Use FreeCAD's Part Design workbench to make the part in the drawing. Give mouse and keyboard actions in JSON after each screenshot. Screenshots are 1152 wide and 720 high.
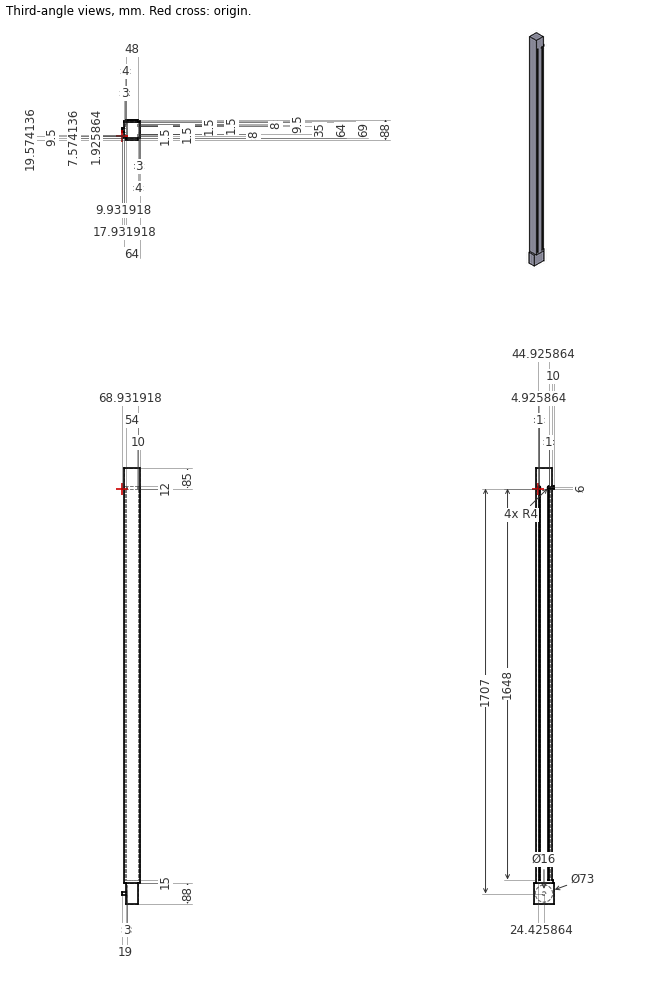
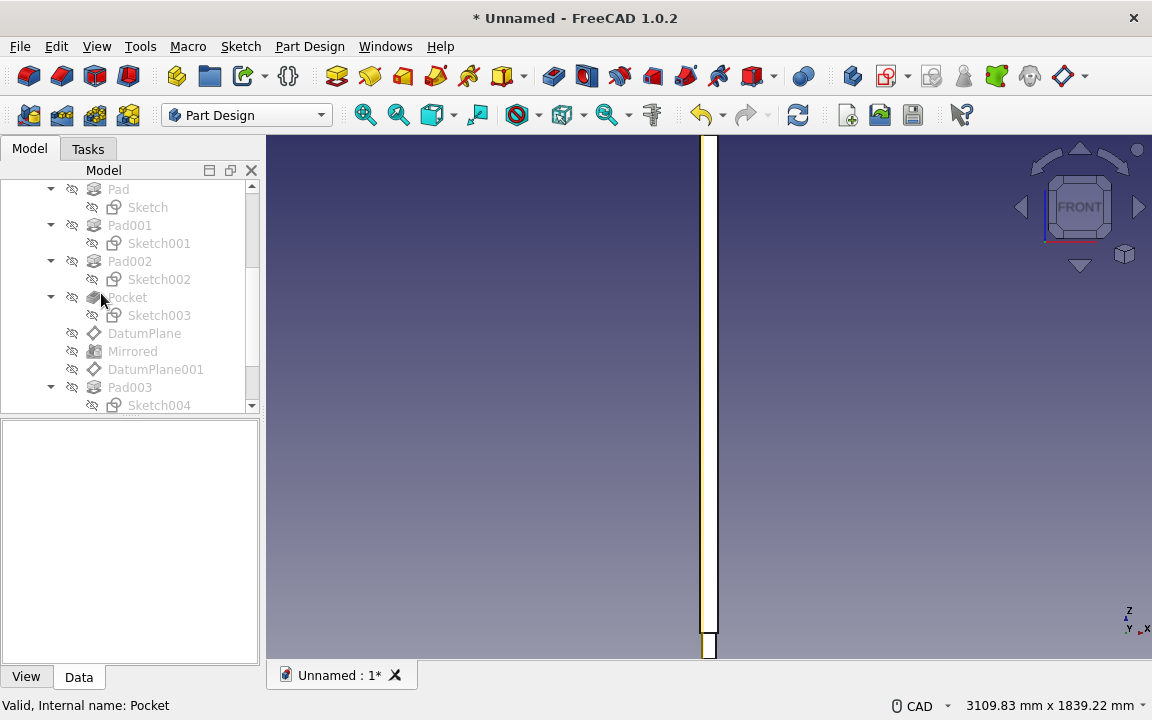
{"action": "scroll", "coordinate": [141, 293], "scroll_direction": "up", "scroll_amount": 15}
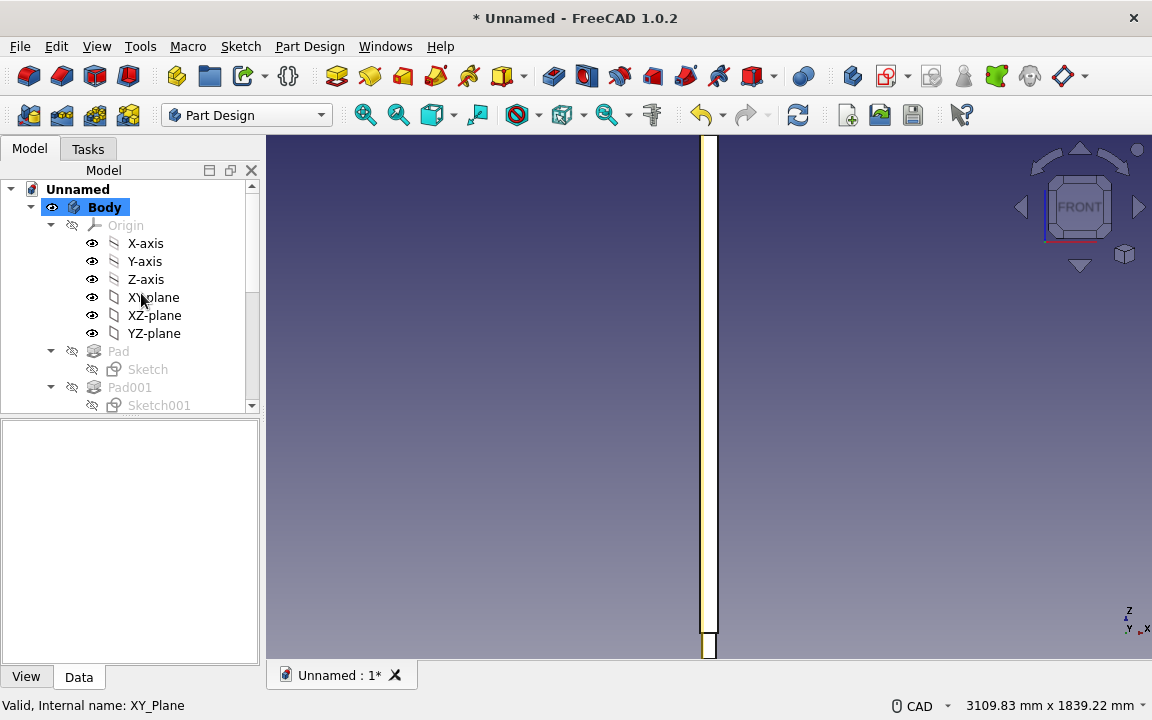
{"action": "scroll", "coordinate": [101, 293], "scroll_direction": "down", "scroll_amount": 6}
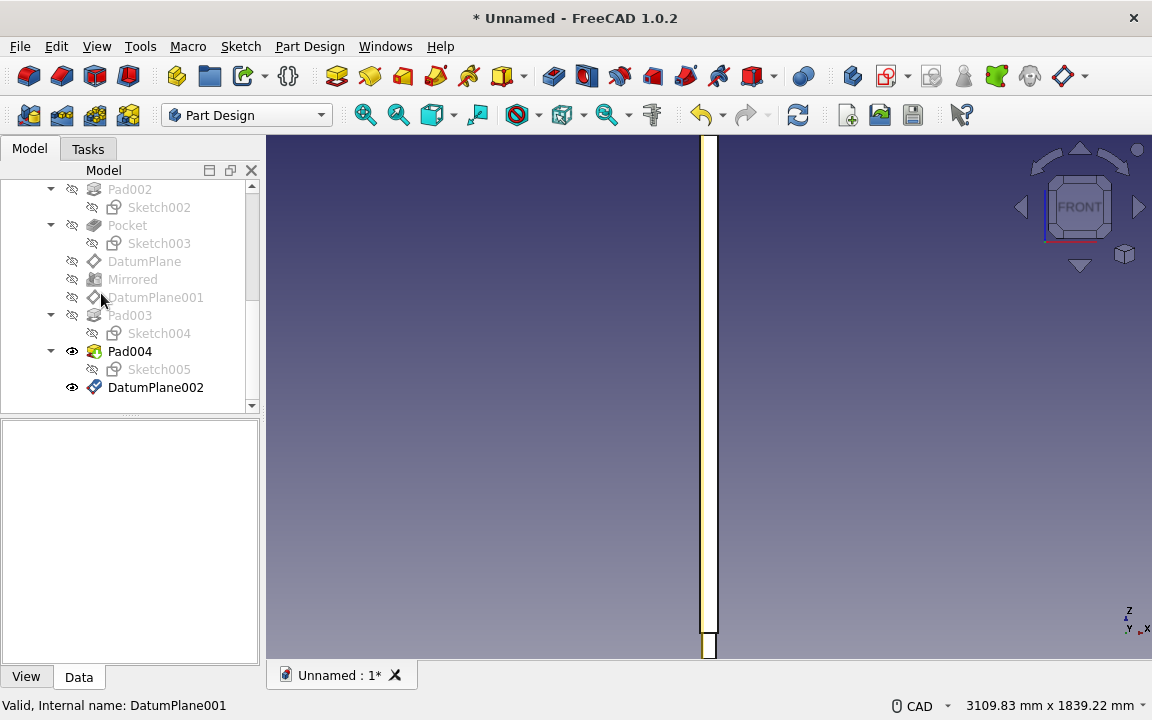
{"action": "left_click", "coordinate": [117, 387]}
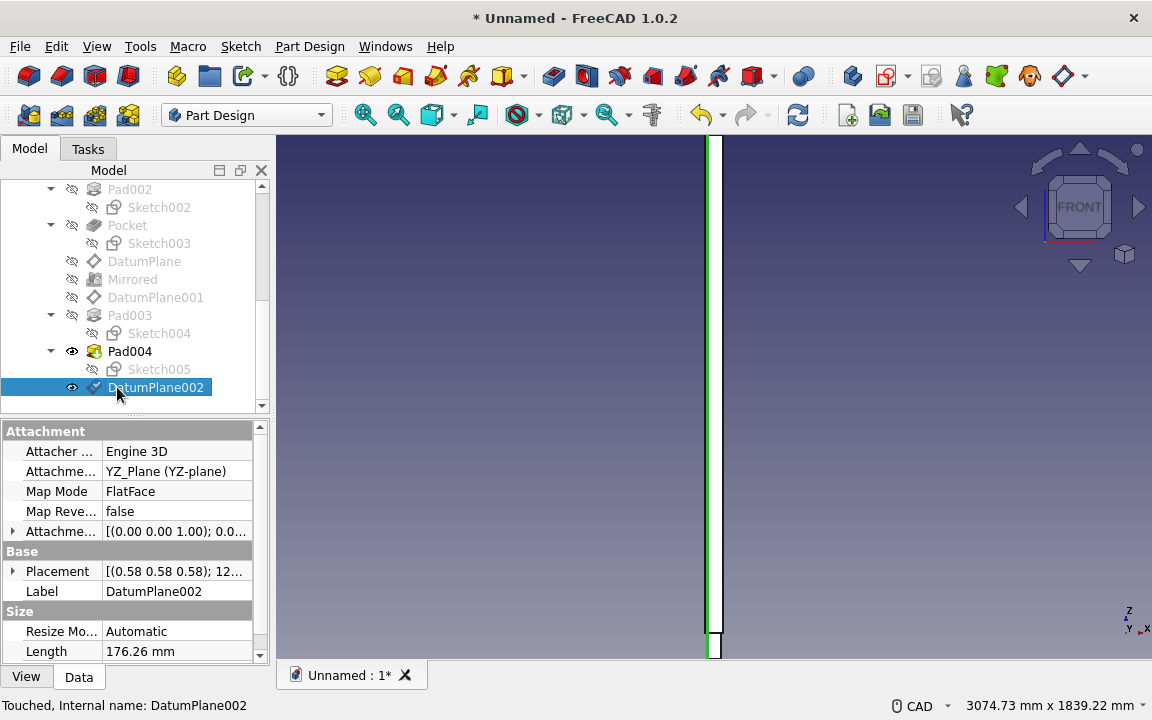
{"action": "left_click", "coordinate": [886, 76]}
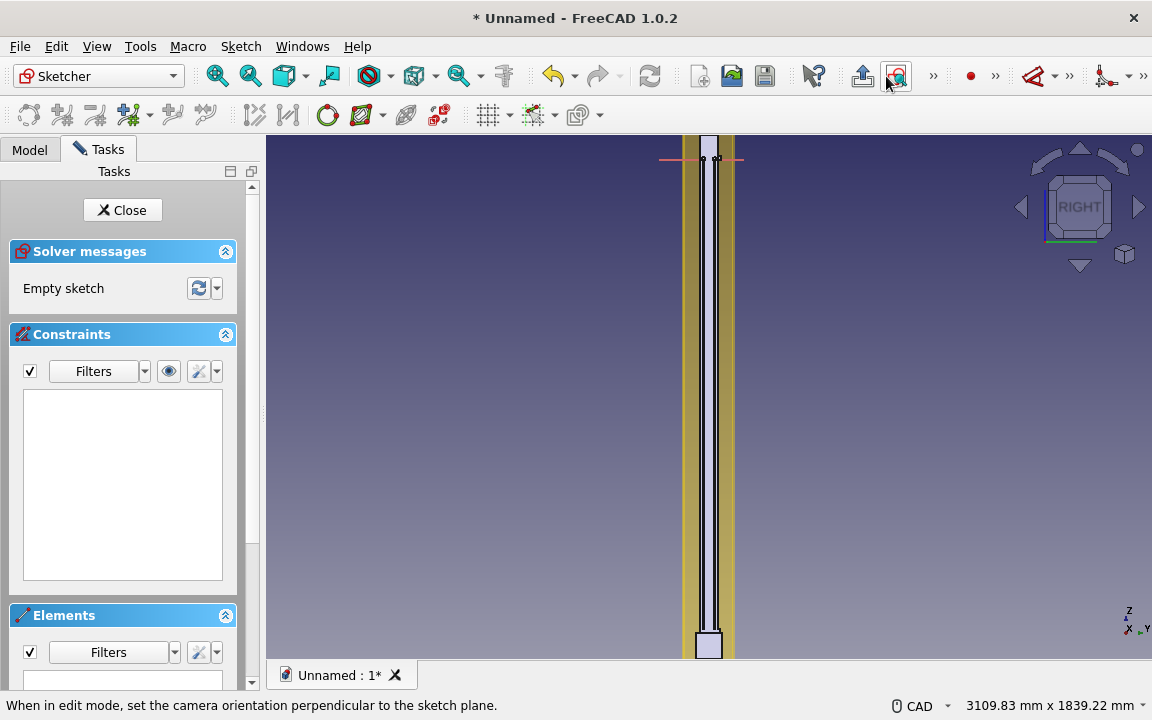
{"action": "key", "text": "q s"}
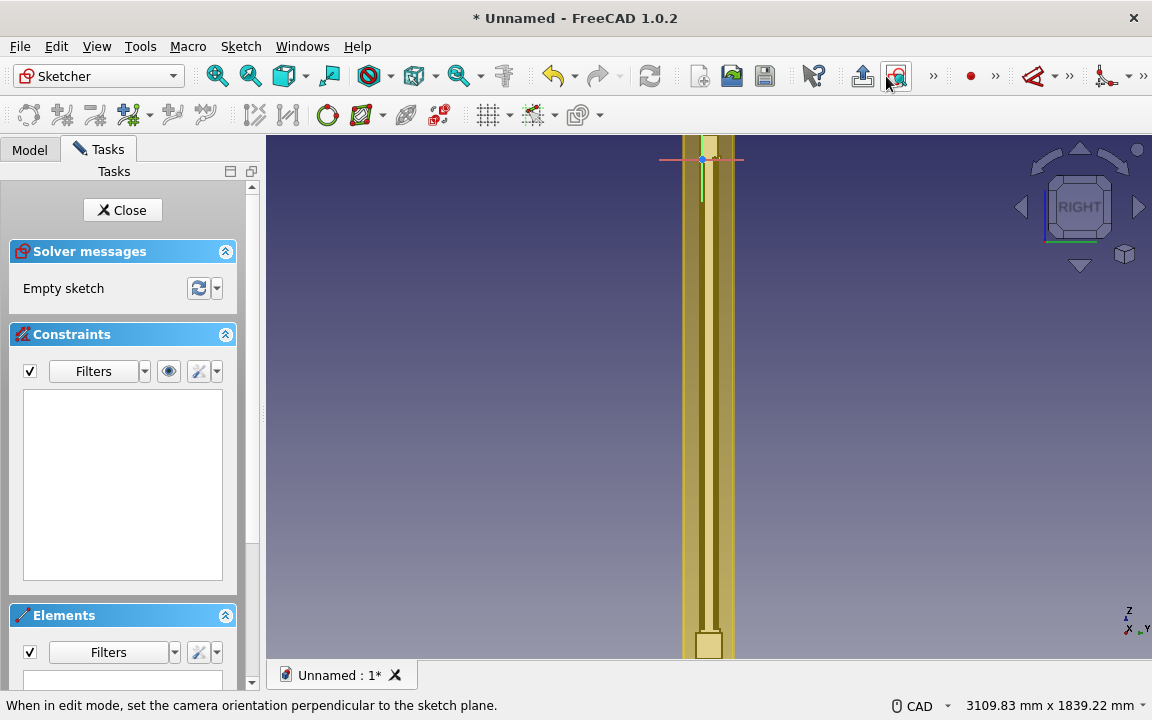
{"action": "scroll", "coordinate": [640, 397], "scroll_direction": "down", "scroll_amount": 5}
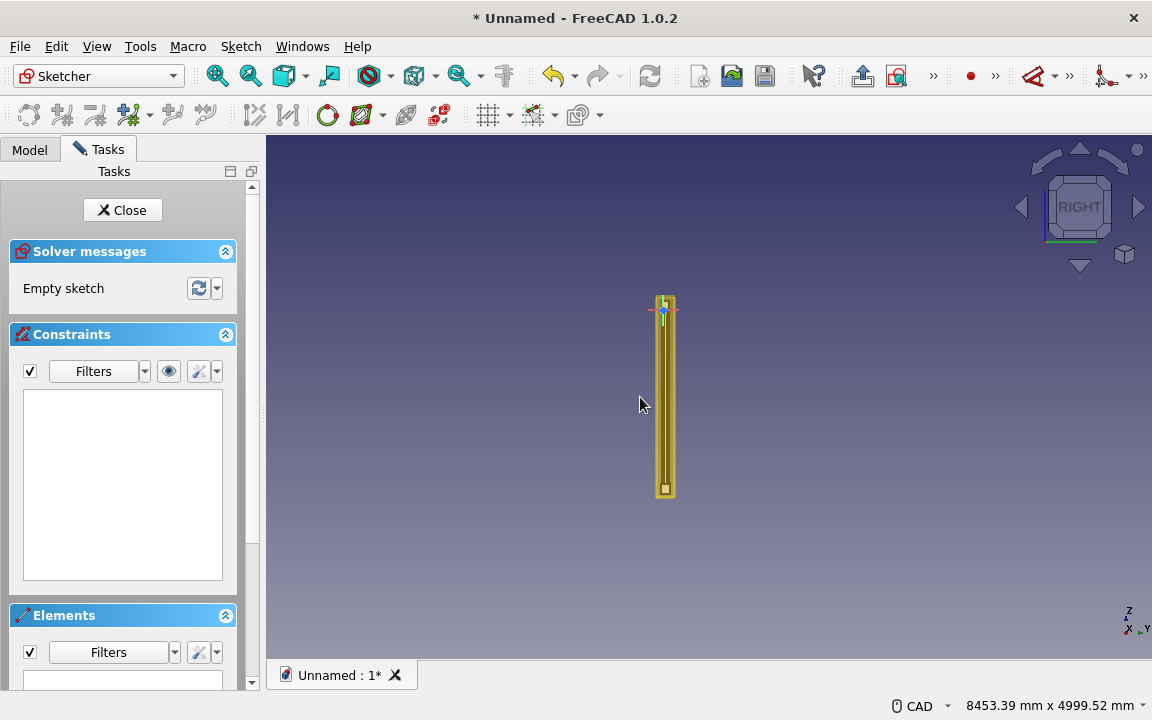
{"action": "scroll", "coordinate": [667, 494], "scroll_direction": "up", "scroll_amount": 15}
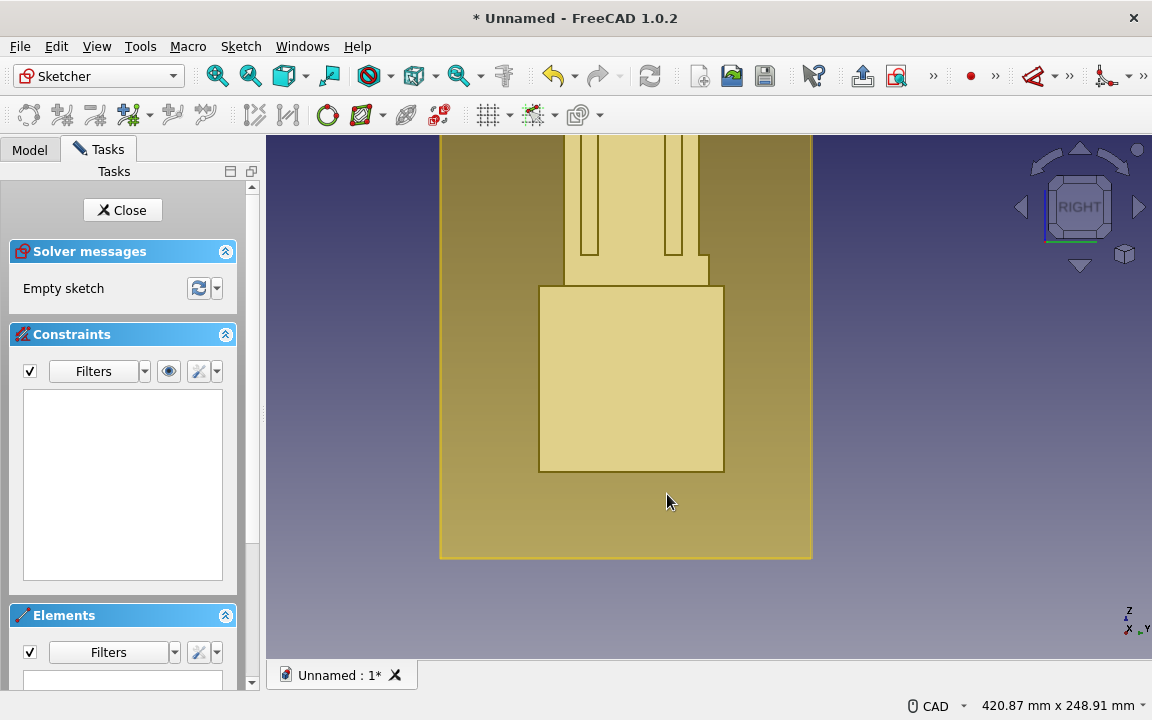
{"action": "scroll", "coordinate": [624, 364], "scroll_direction": "up", "scroll_amount": 4}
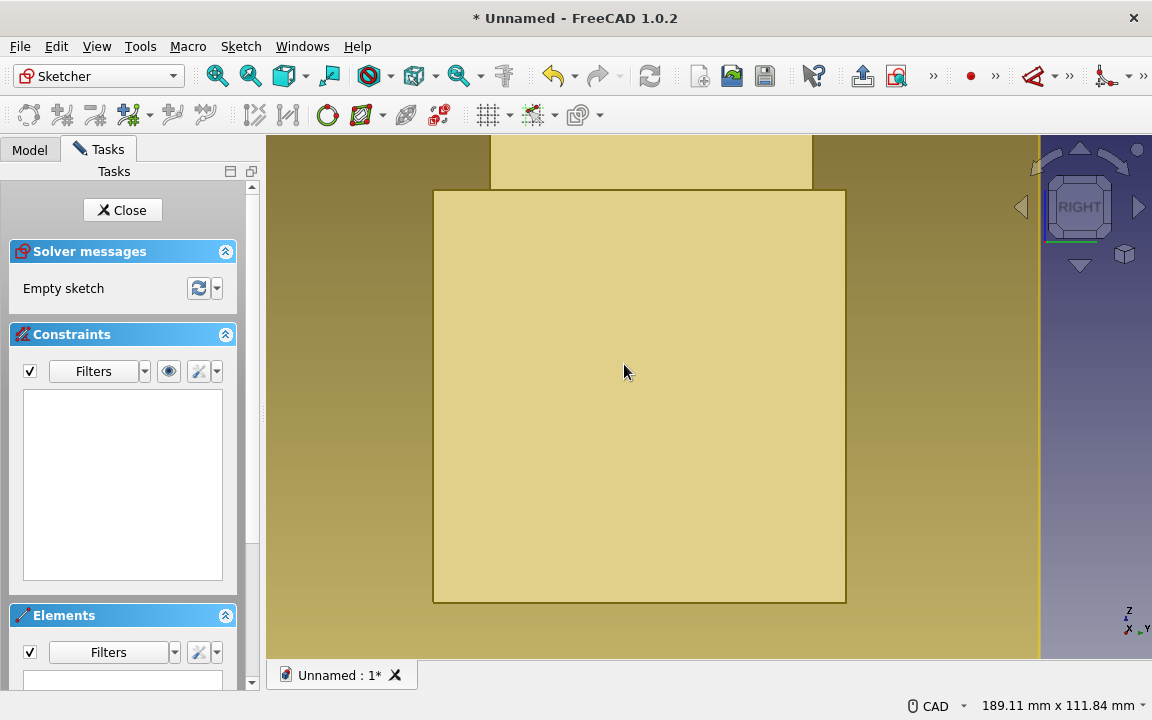
{"action": "key", "text": "g c"}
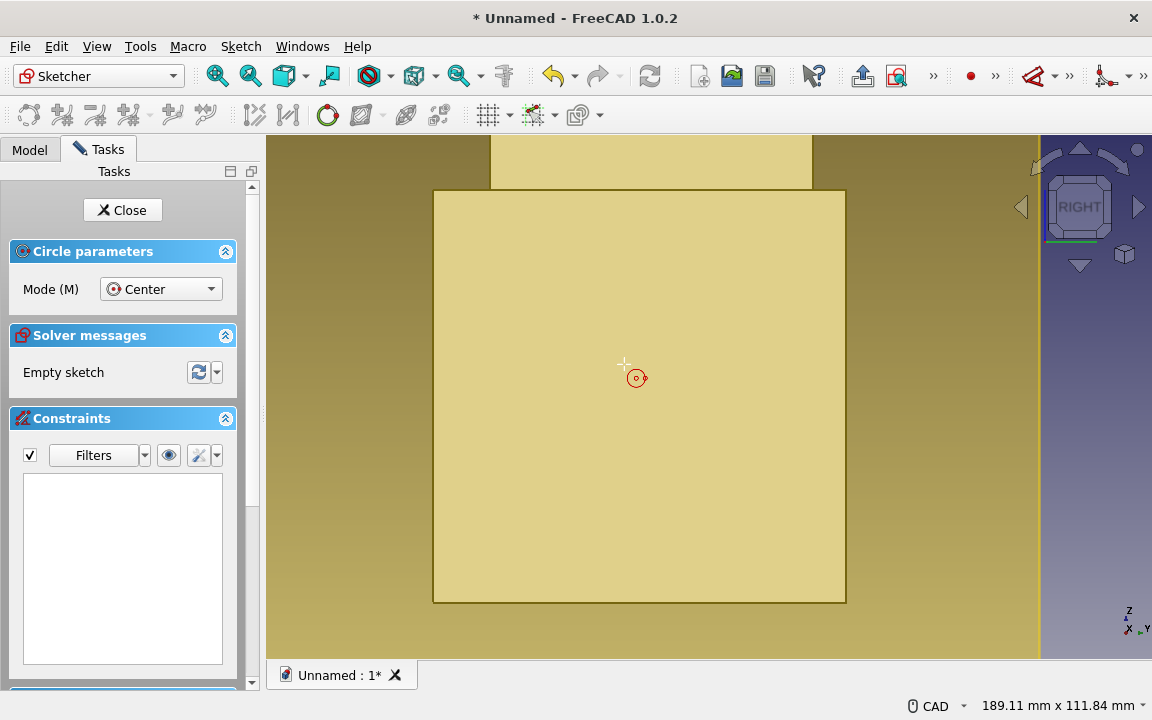
{"action": "left_click", "coordinate": [640, 397]}
{"action": "mouse_move", "coordinate": [761, 276]}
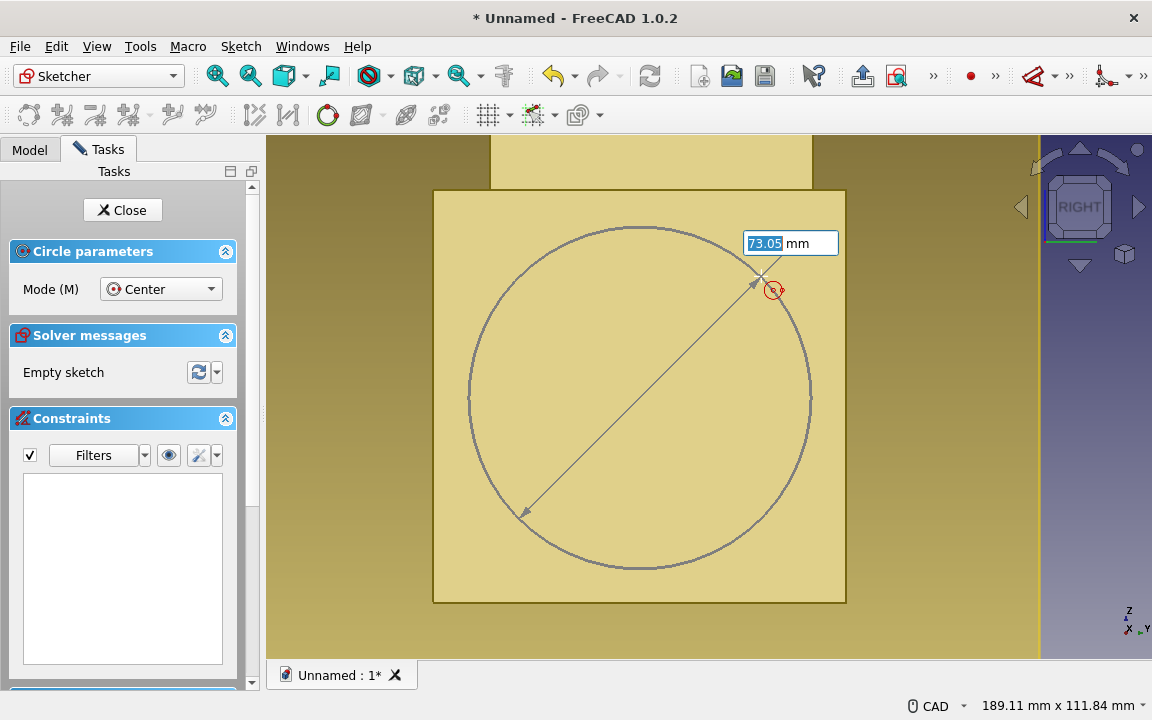
{"action": "type", "text": "73"}
{"action": "key", "text": "Return"}
{"action": "key", "text": "Escape"}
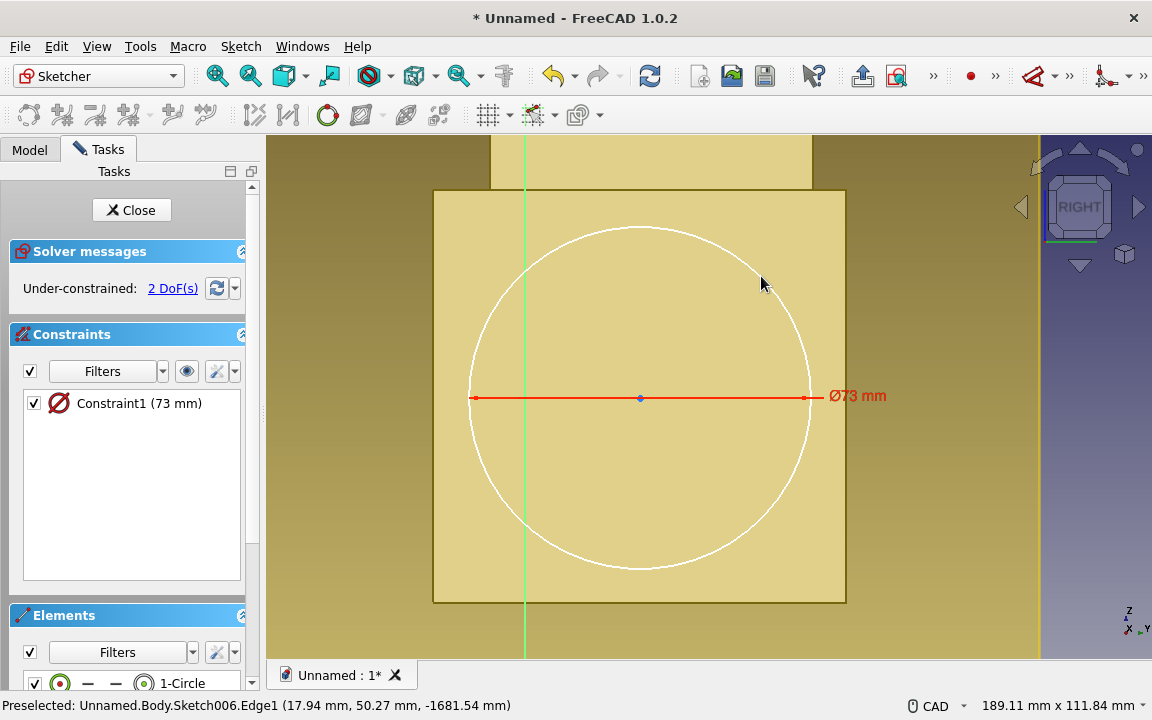
{"action": "left_click", "coordinate": [1032, 76]}